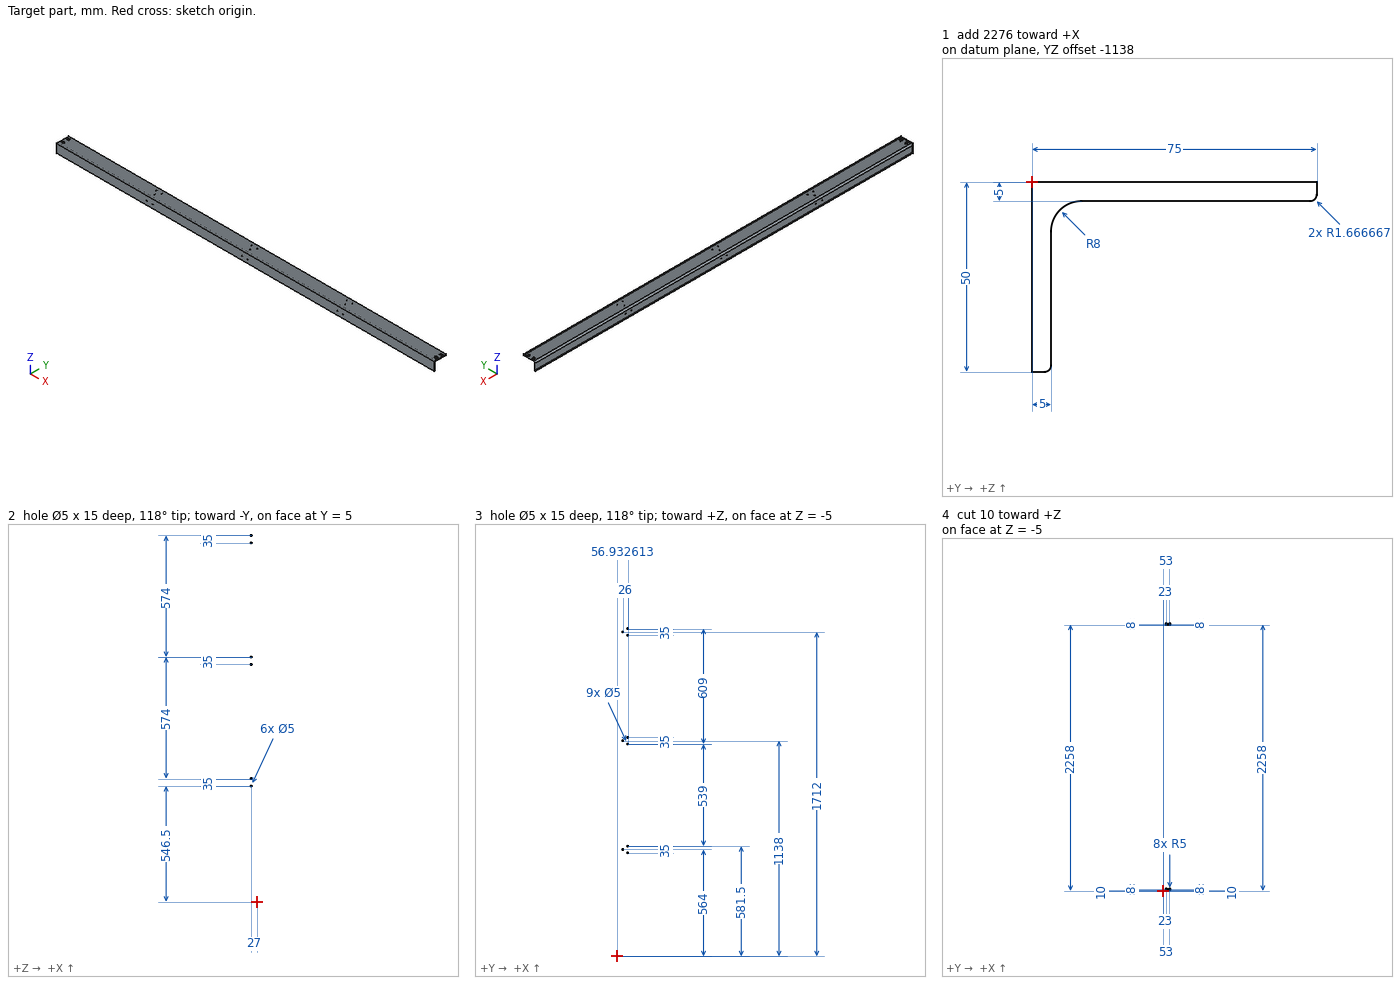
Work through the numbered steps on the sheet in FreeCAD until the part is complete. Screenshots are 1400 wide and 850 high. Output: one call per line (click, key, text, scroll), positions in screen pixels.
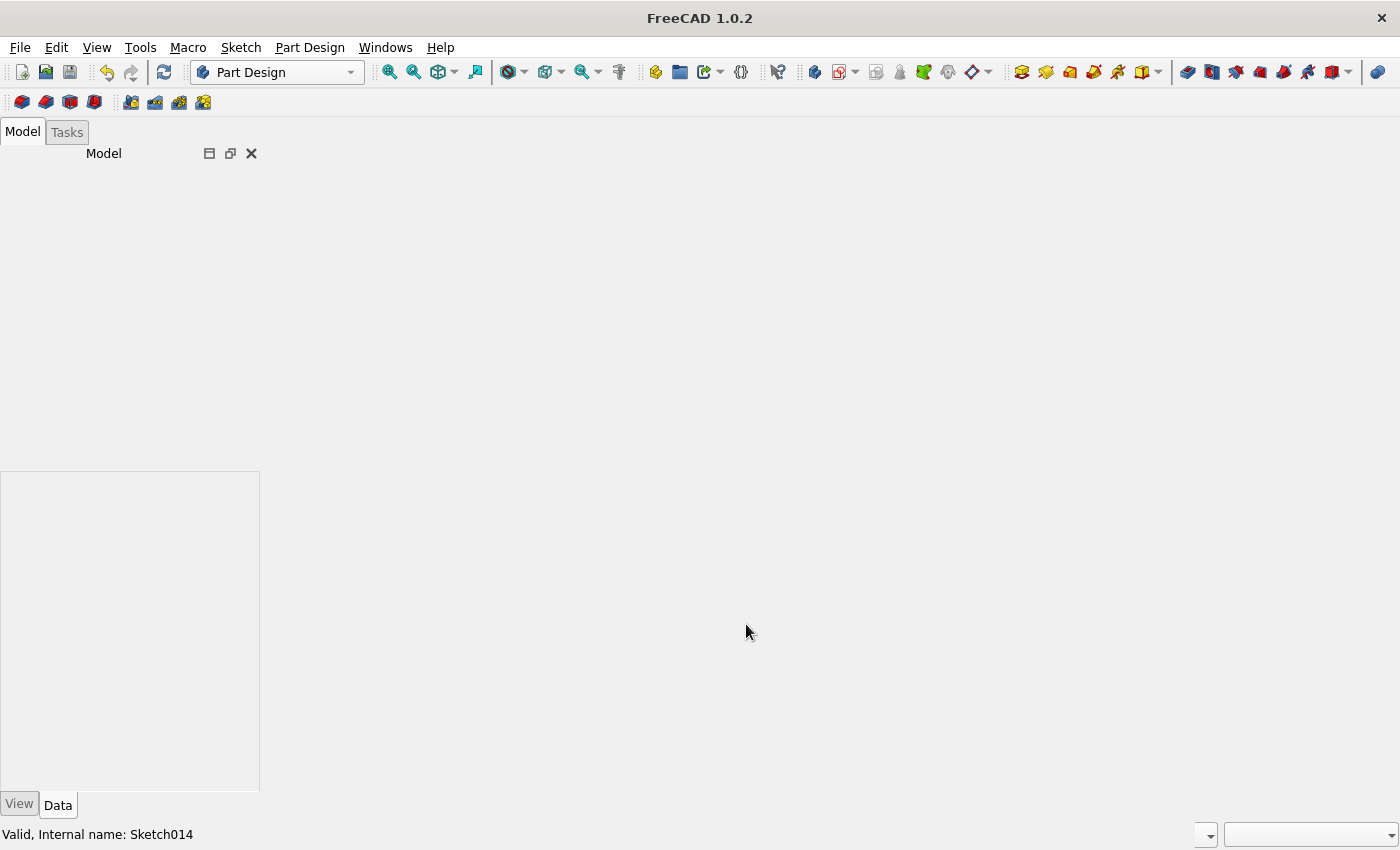
click(22, 72)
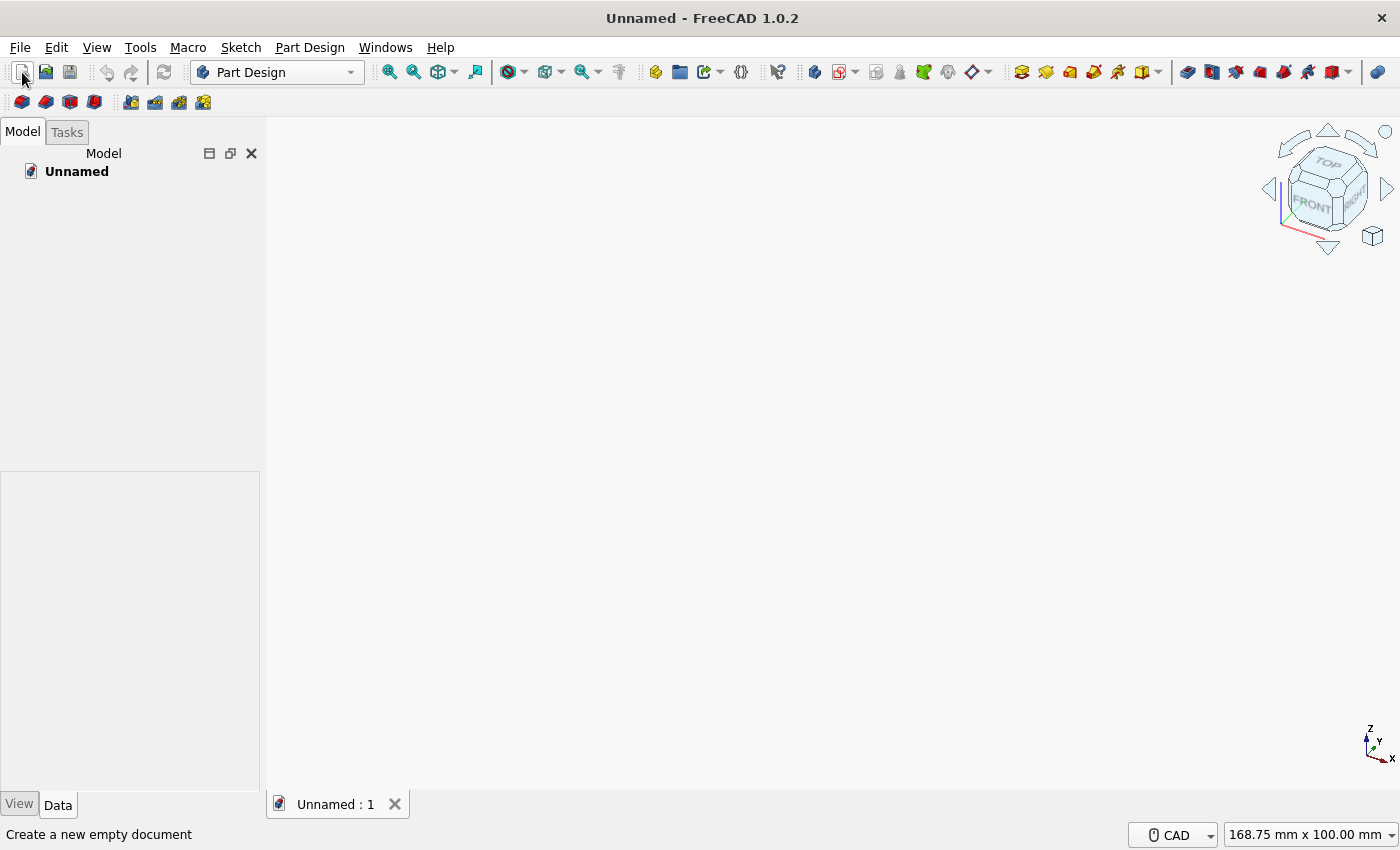
click(816, 72)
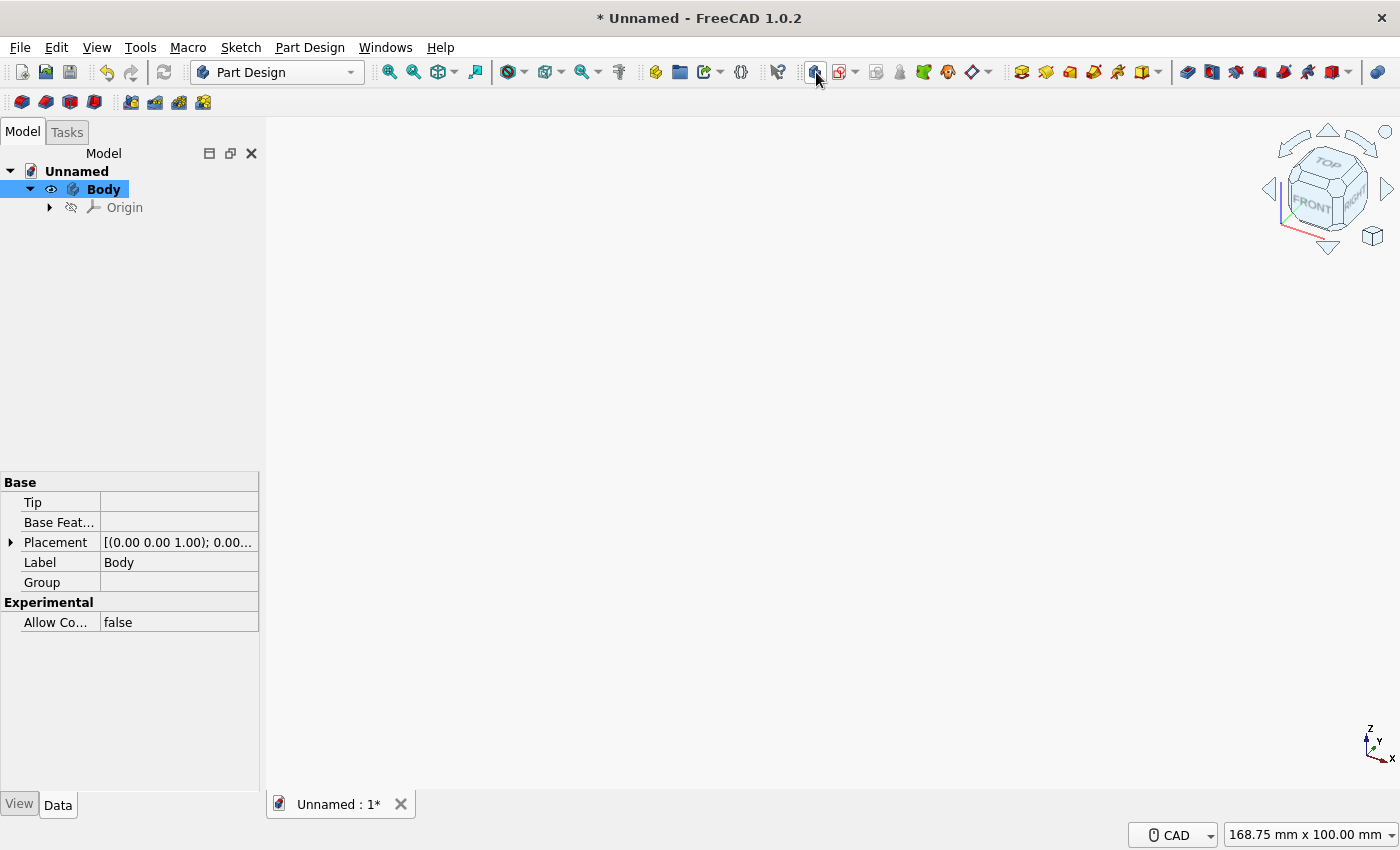
click(50, 207)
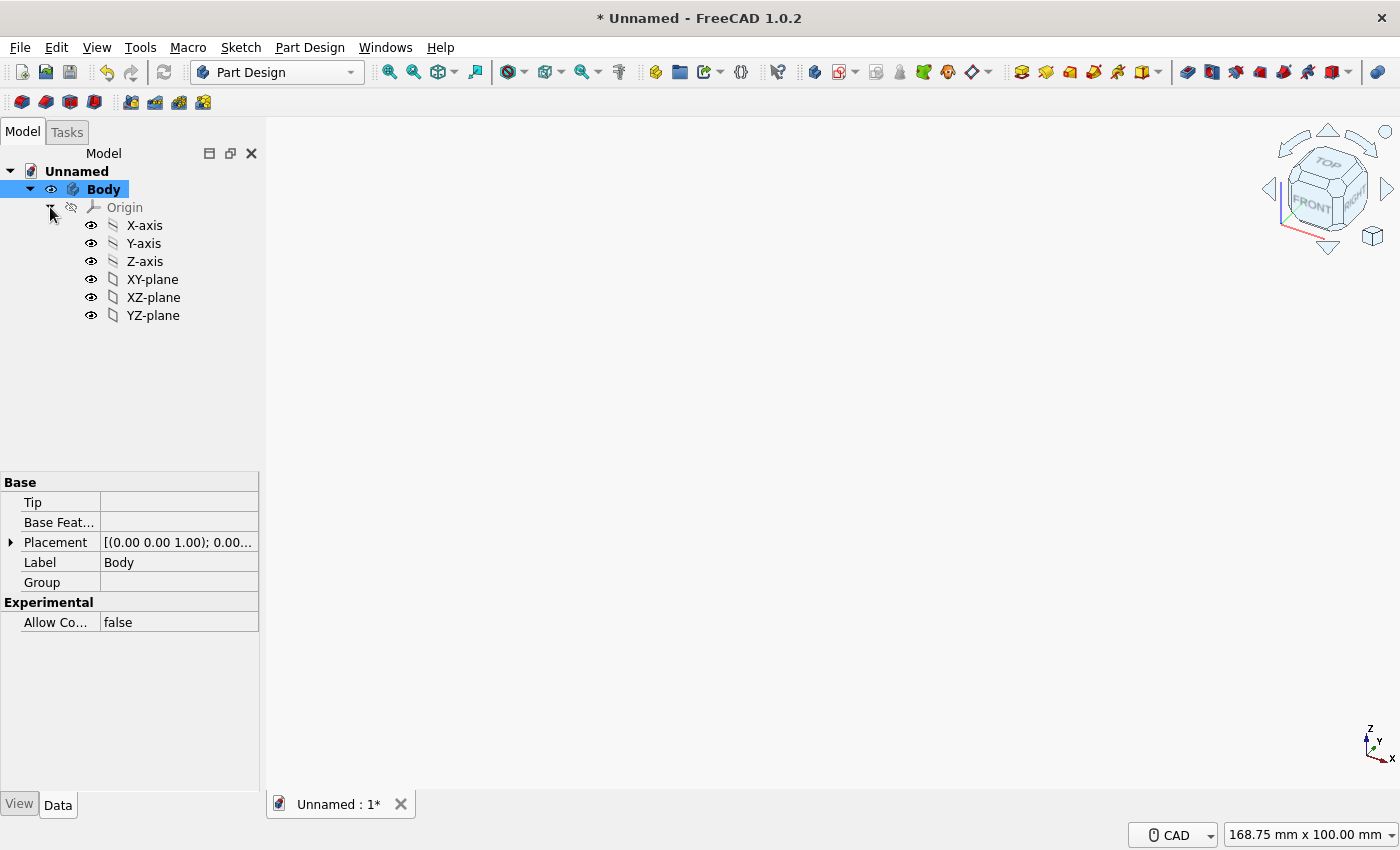
click(136, 315)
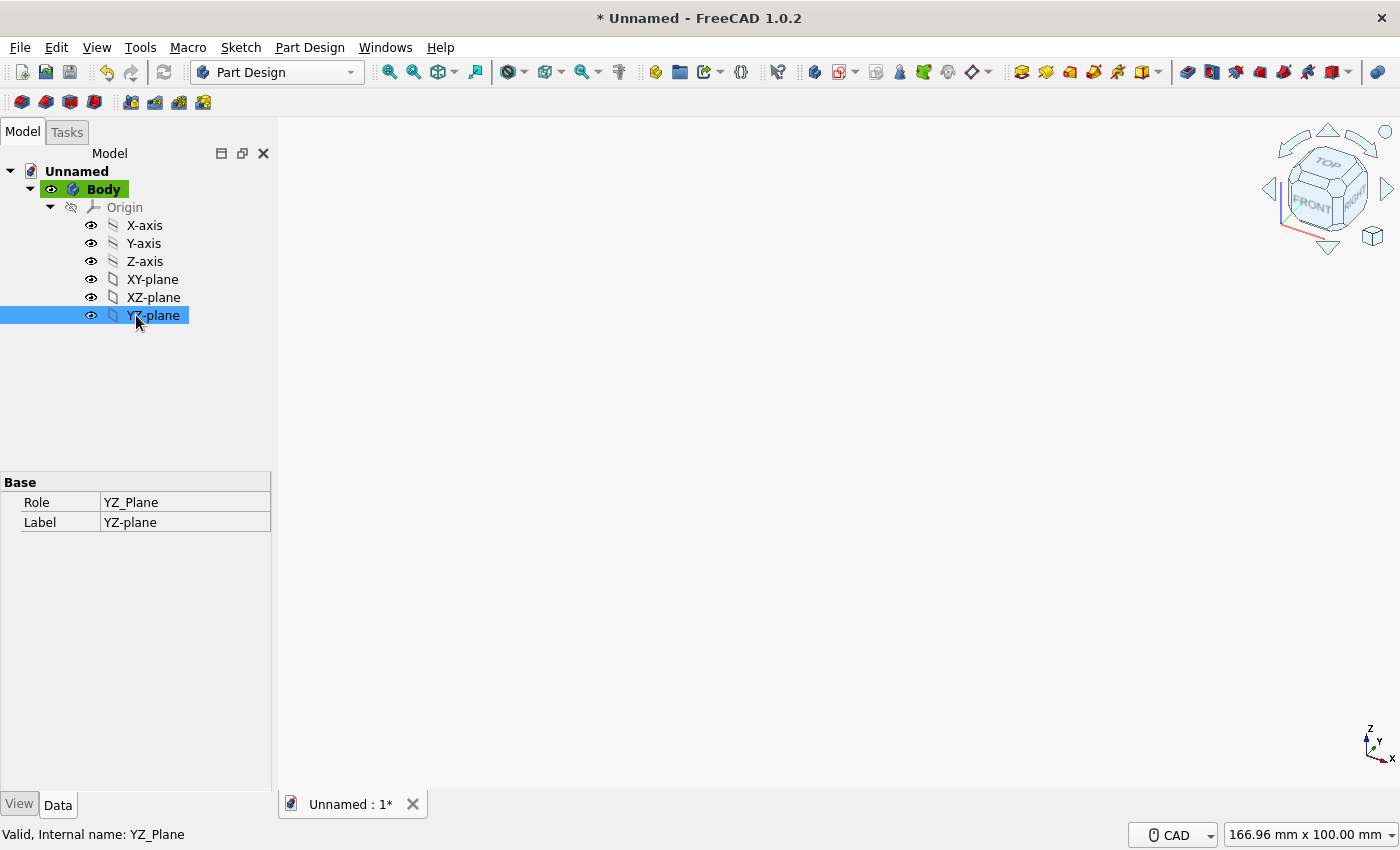
click(972, 72)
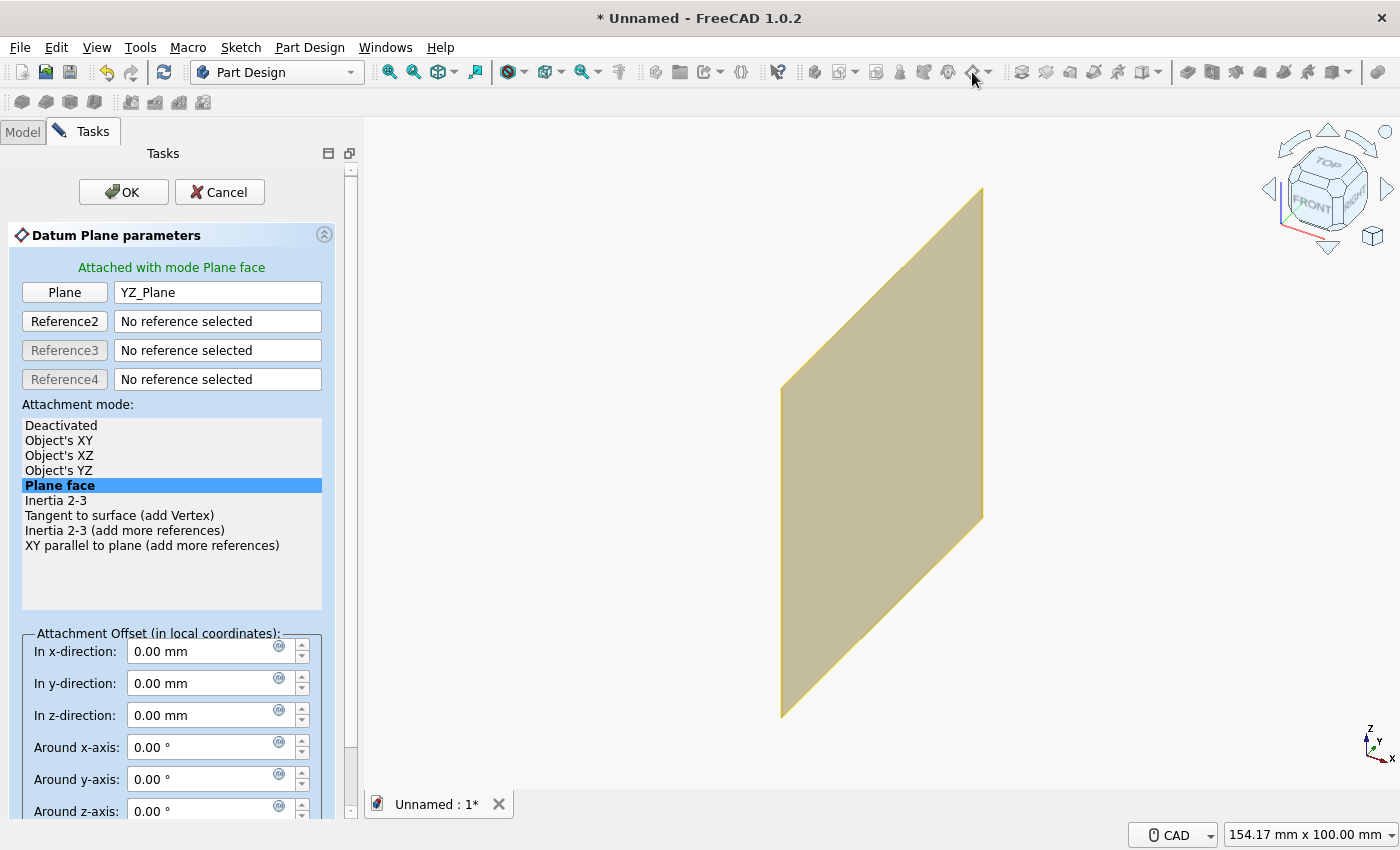
triple_click(210, 715)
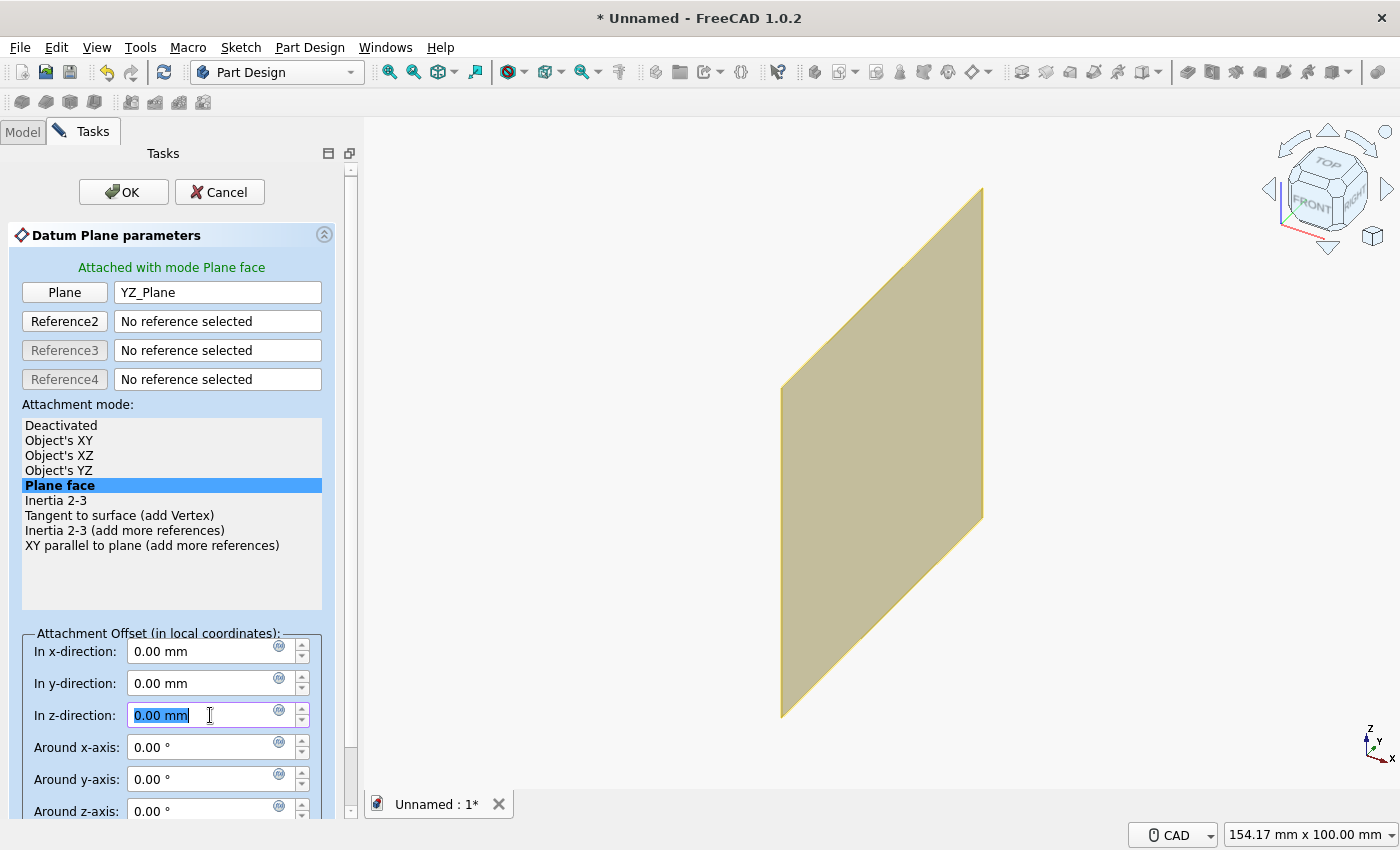
text(-1138)
key(Tab)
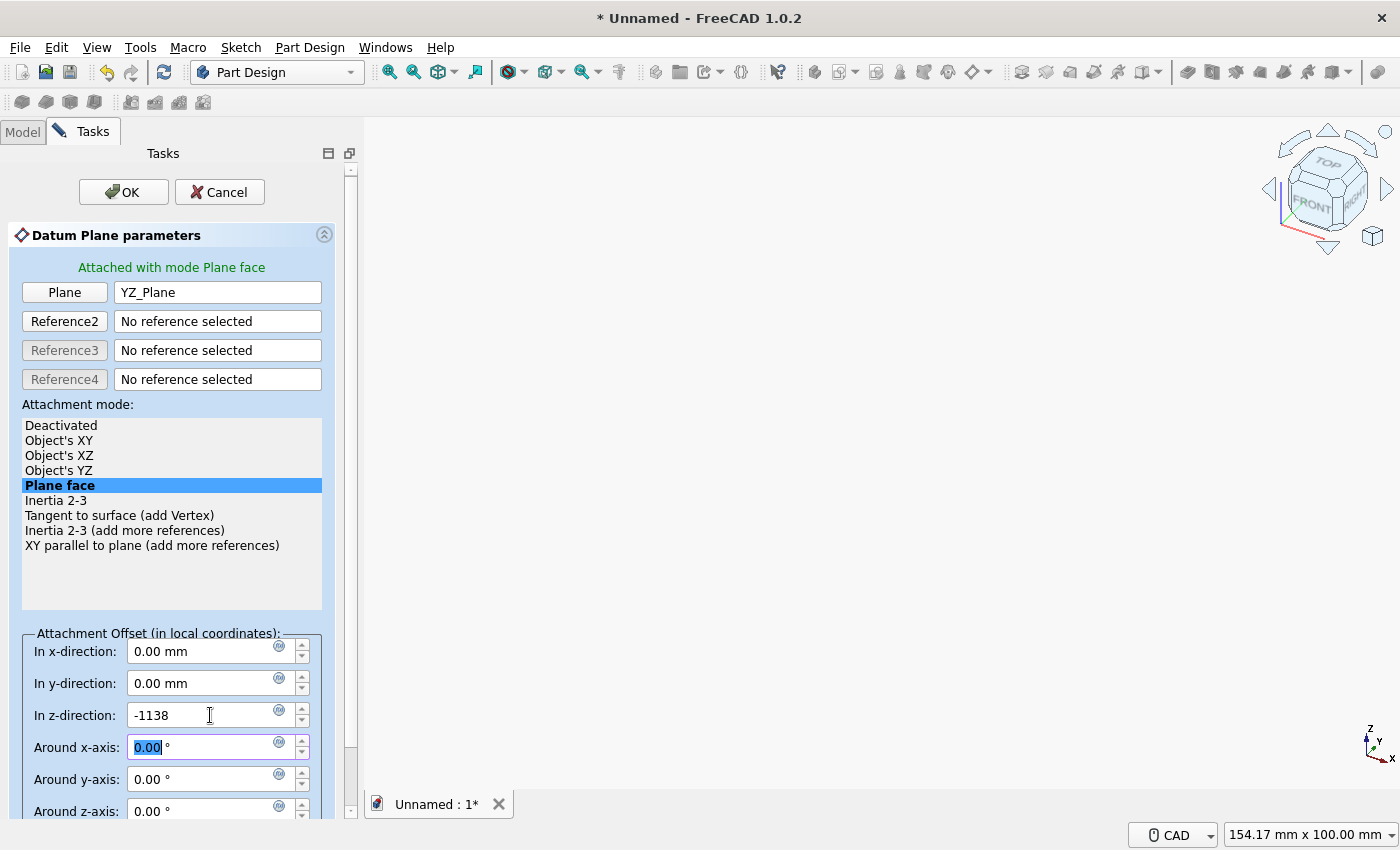
click(124, 192)